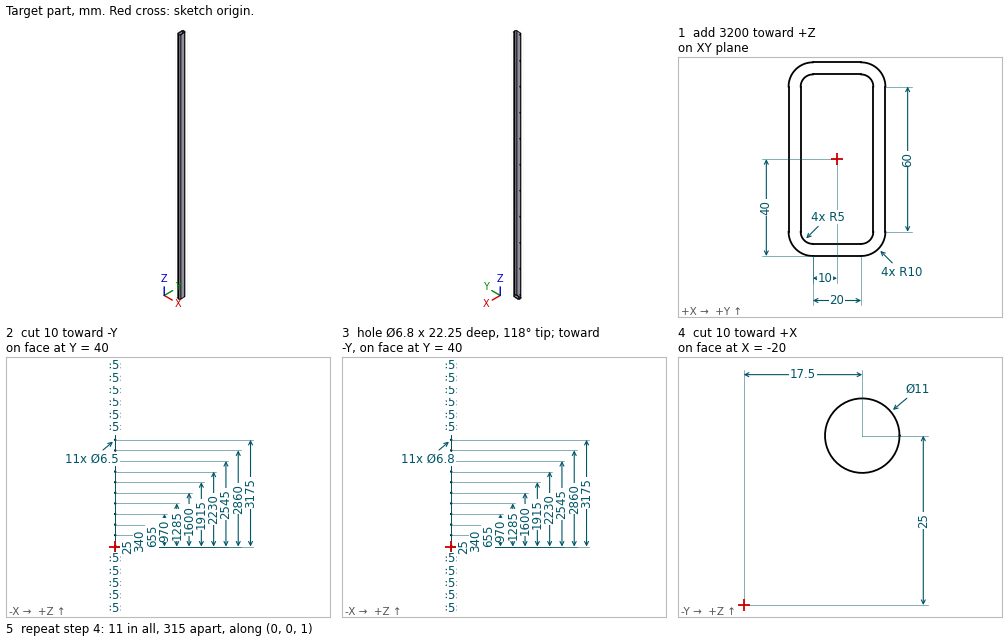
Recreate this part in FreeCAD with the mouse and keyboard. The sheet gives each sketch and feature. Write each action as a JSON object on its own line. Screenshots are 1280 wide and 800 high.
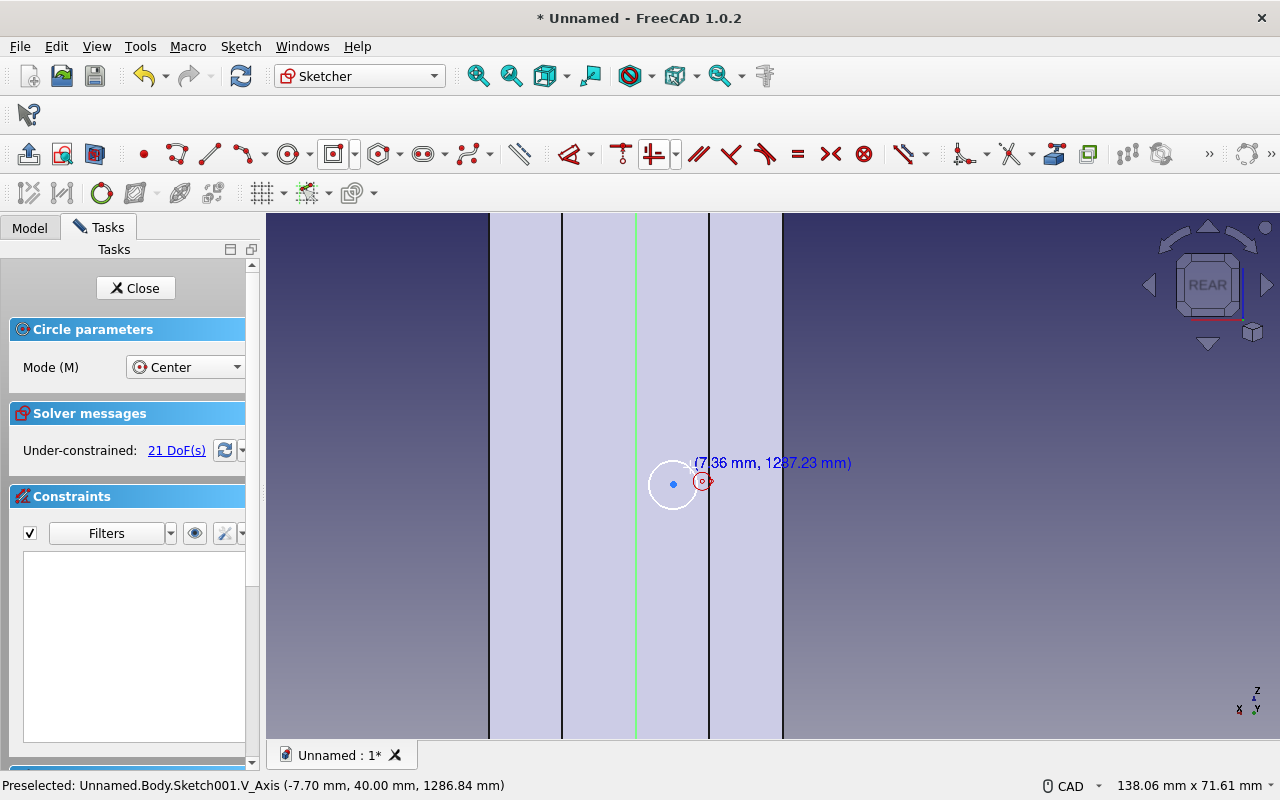
{"action": "scroll", "coordinate": [704, 476], "scroll_direction": "down", "scroll_amount": 15}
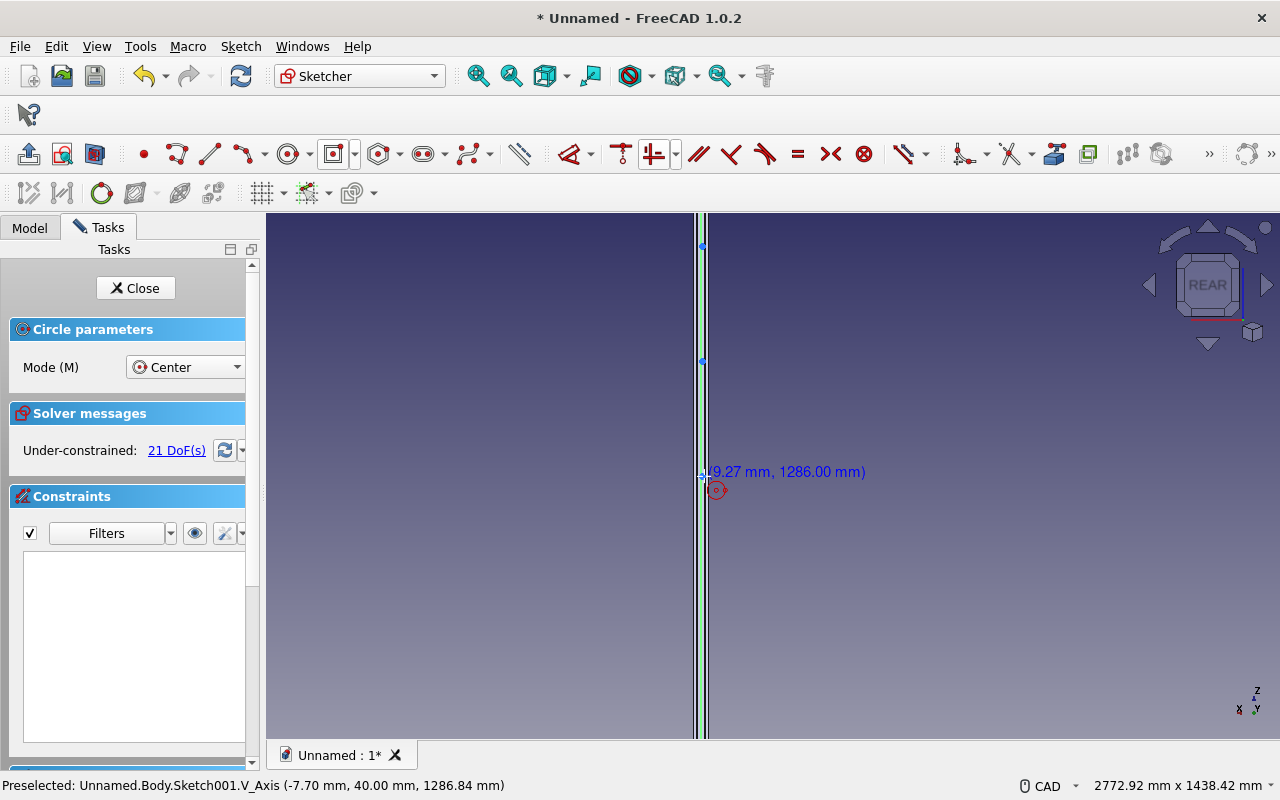
{"action": "scroll", "coordinate": [705, 524], "scroll_direction": "down", "scroll_amount": 6}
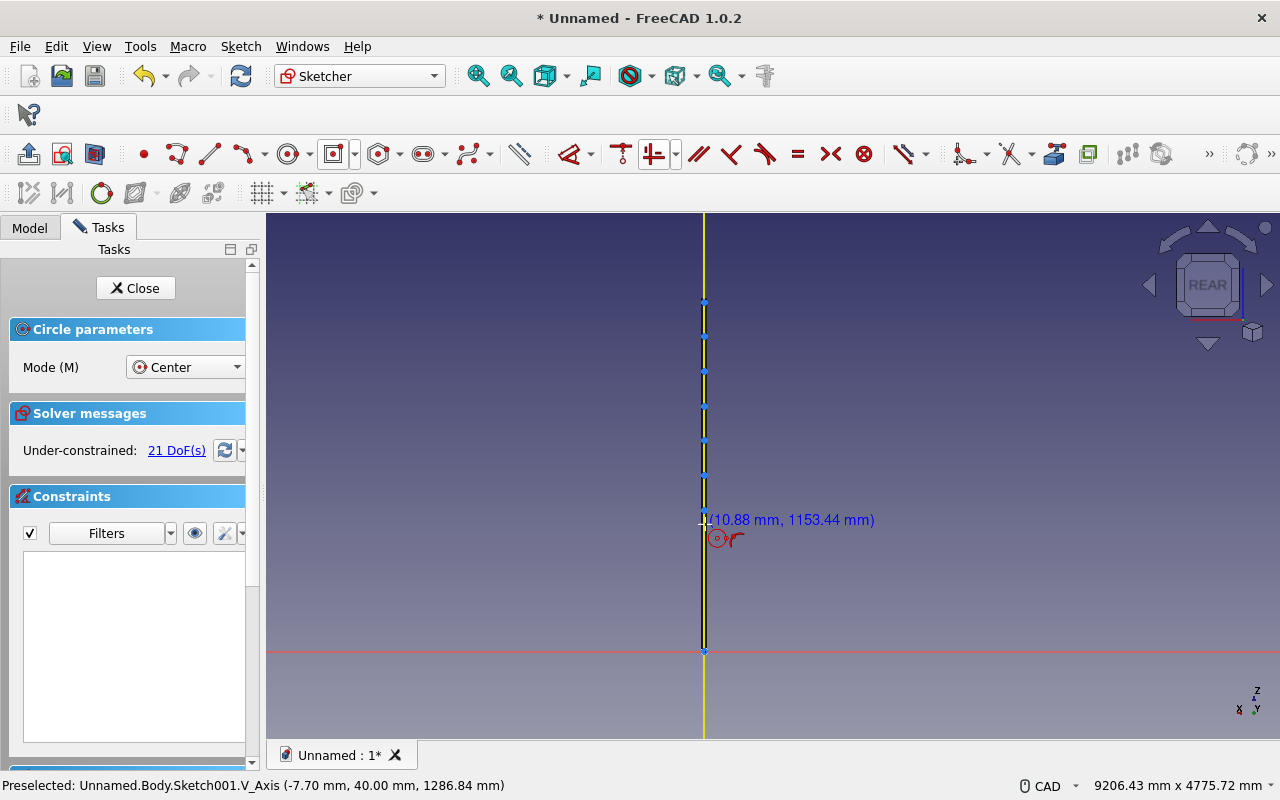
{"action": "scroll", "coordinate": [705, 545], "scroll_direction": "up", "scroll_amount": 21}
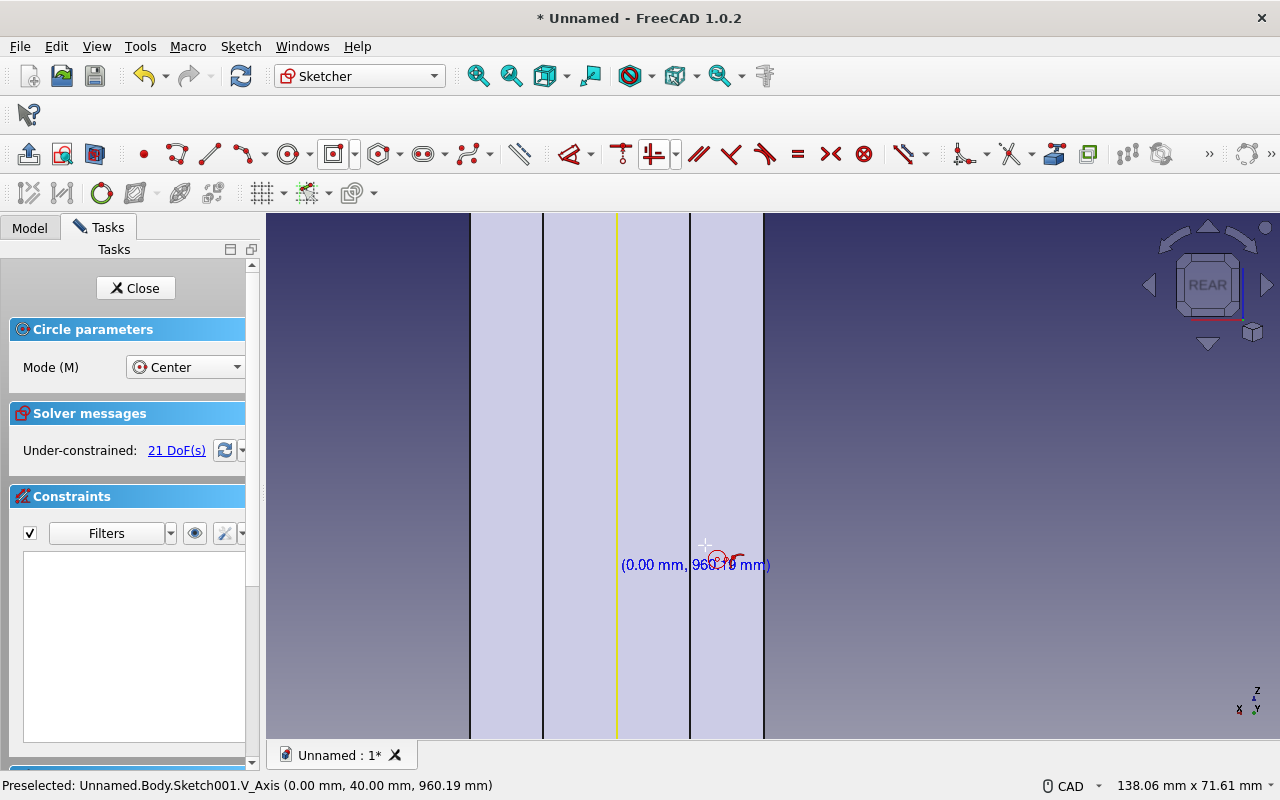
{"action": "left_click", "coordinate": [654, 498]}
{"action": "left_click", "coordinate": [670, 481]}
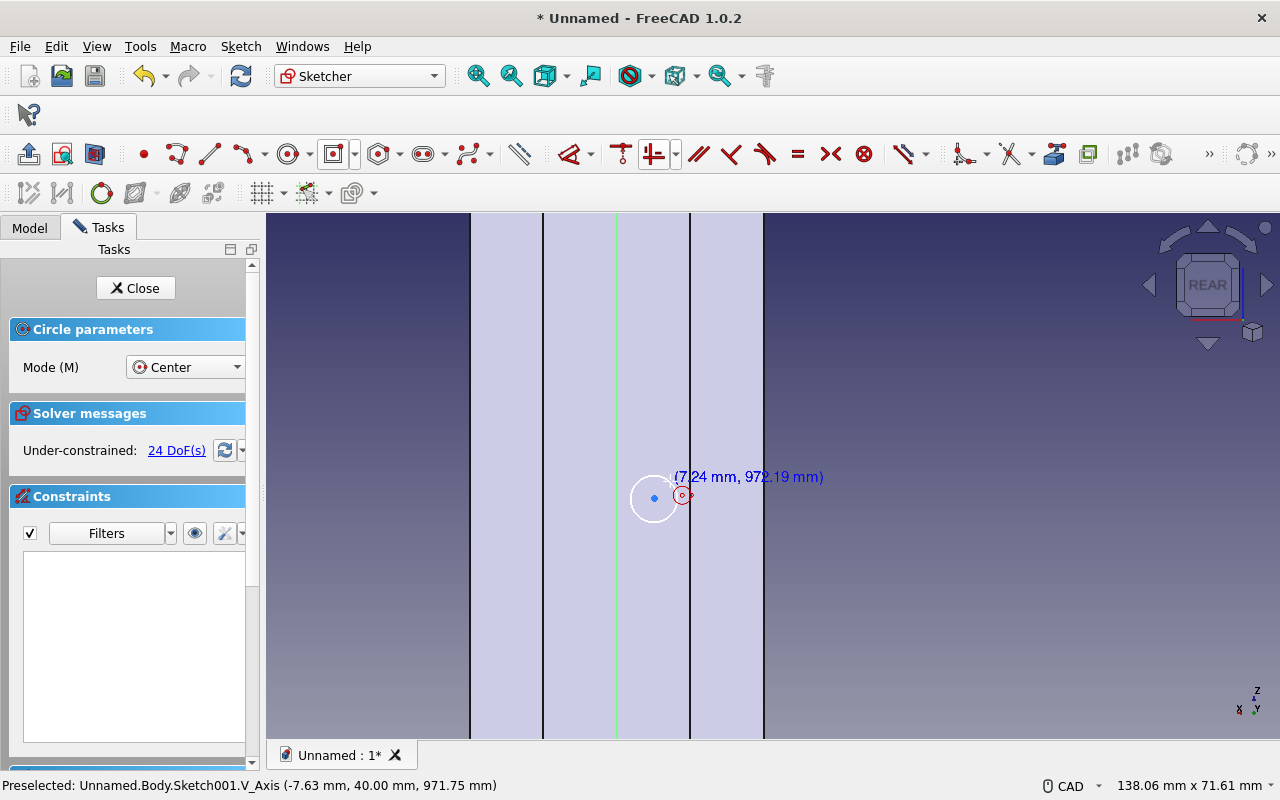
{"action": "scroll", "coordinate": [704, 476], "scroll_direction": "down", "scroll_amount": 15}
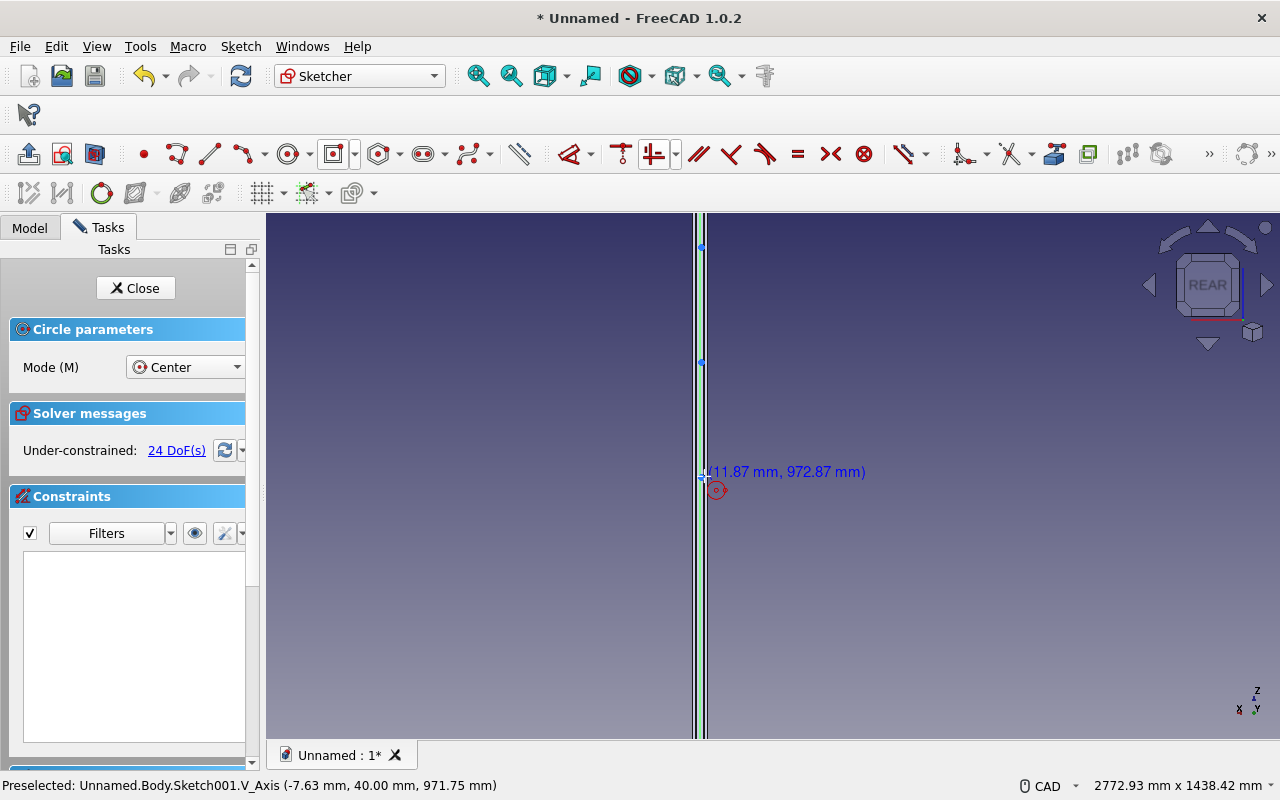
{"action": "scroll", "coordinate": [706, 573], "scroll_direction": "down", "scroll_amount": 6}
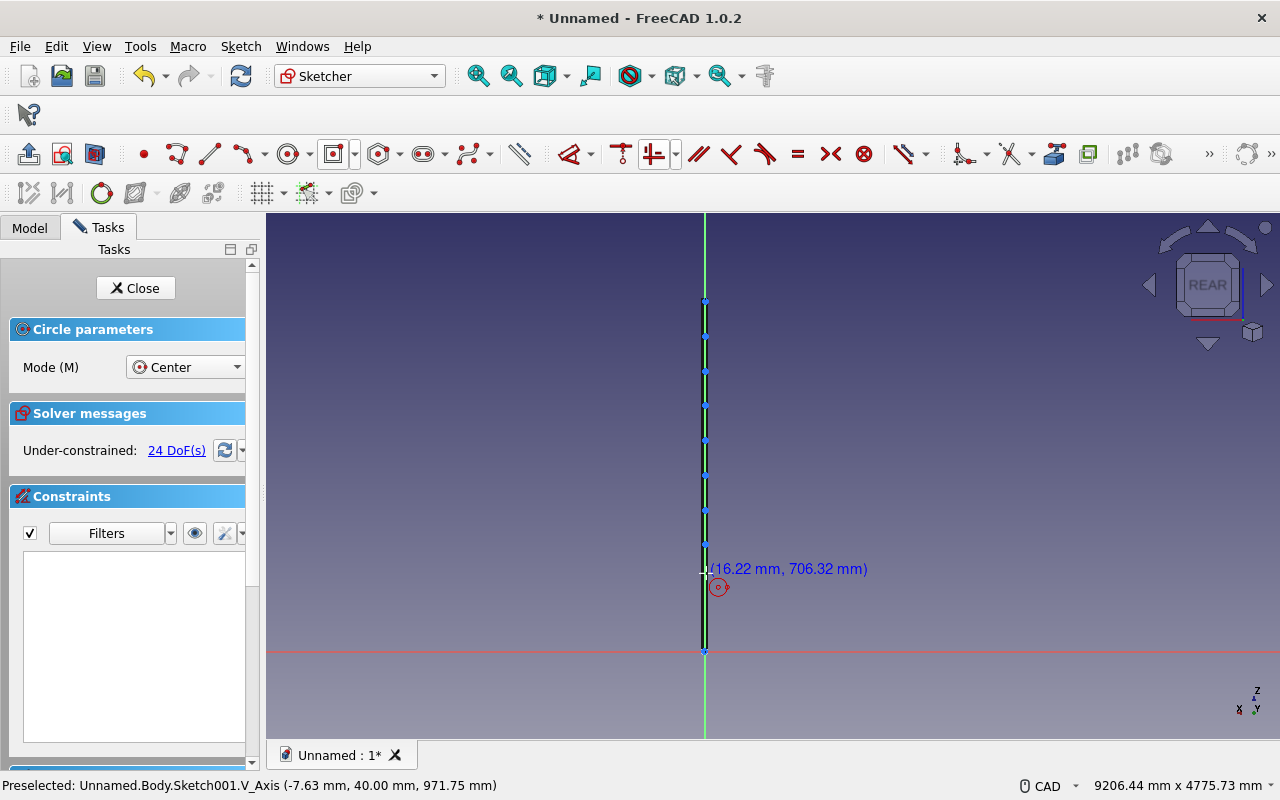
{"action": "scroll", "coordinate": [705, 579], "scroll_direction": "up", "scroll_amount": 21}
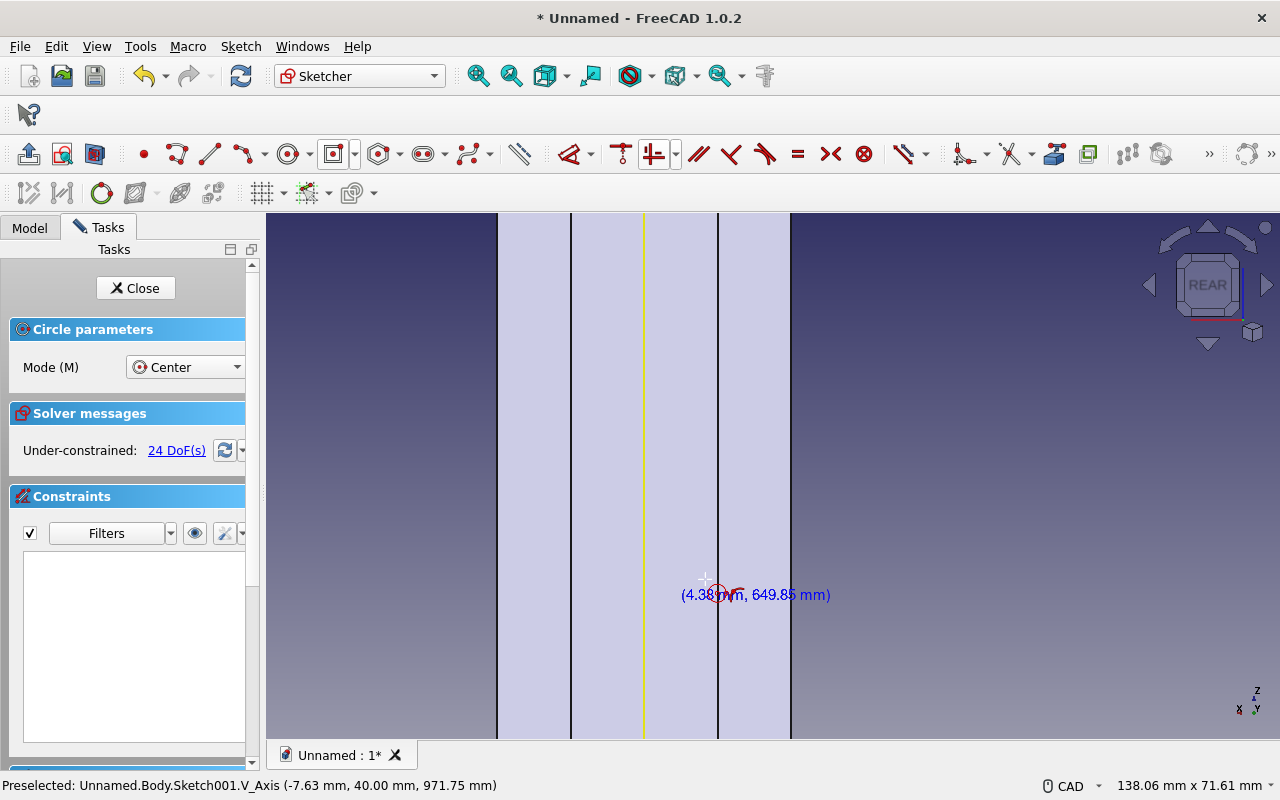
{"action": "left_click", "coordinate": [681, 562]}
{"action": "left_click", "coordinate": [698, 545]}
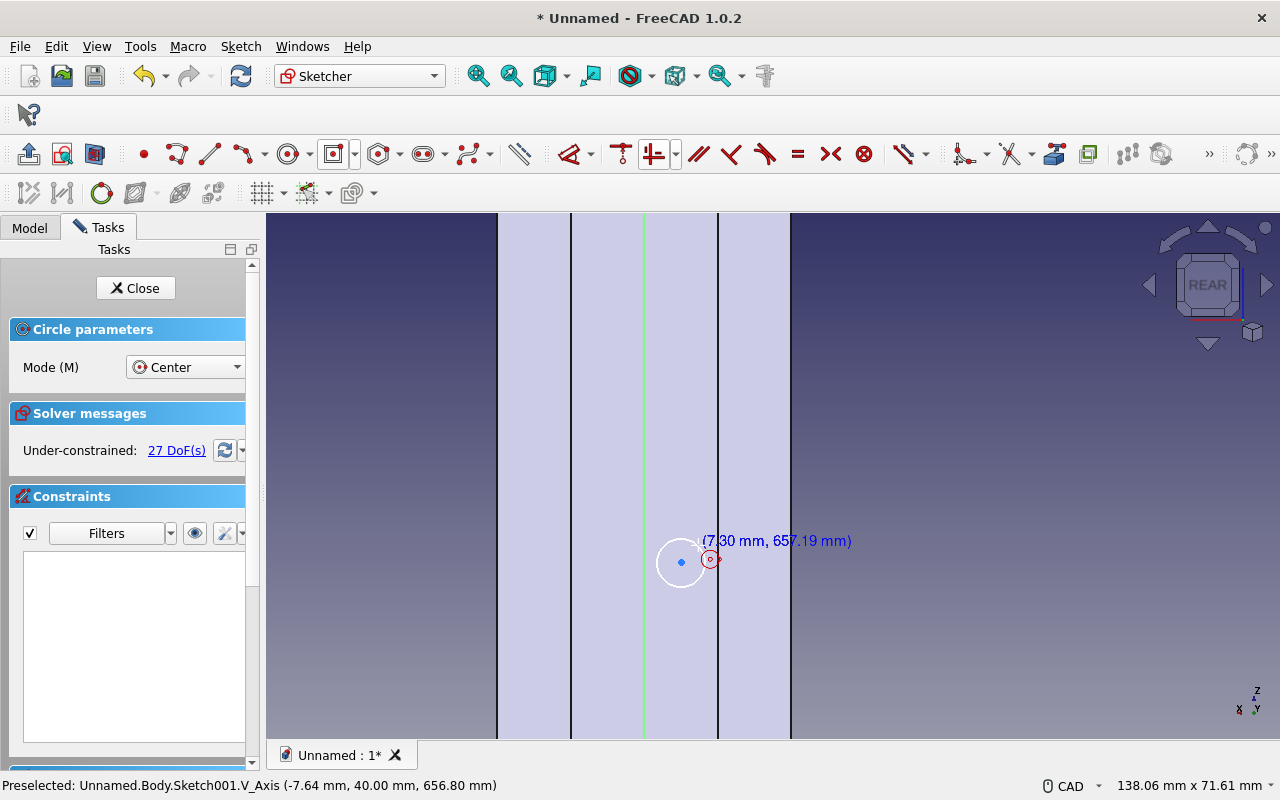
{"action": "scroll", "coordinate": [704, 476], "scroll_direction": "down", "scroll_amount": 15}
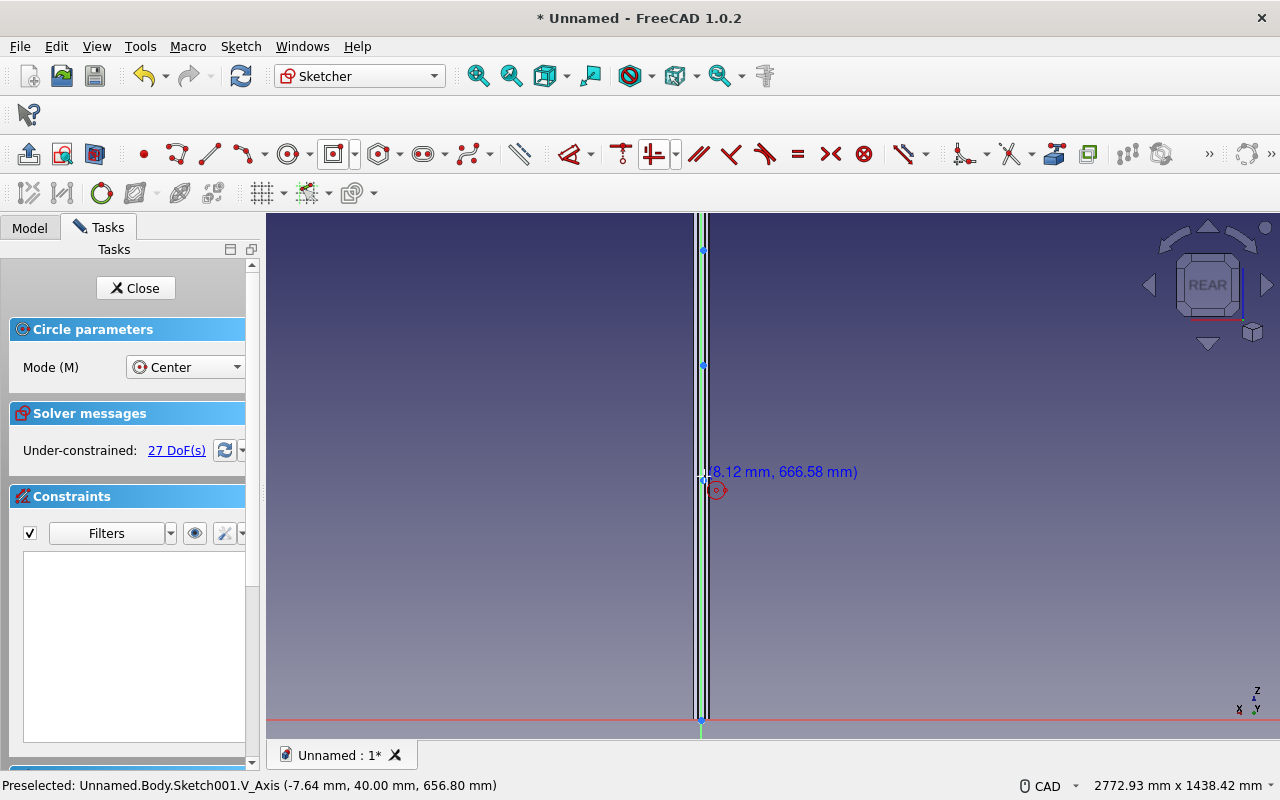
{"action": "scroll", "coordinate": [705, 621], "scroll_direction": "down", "scroll_amount": 6}